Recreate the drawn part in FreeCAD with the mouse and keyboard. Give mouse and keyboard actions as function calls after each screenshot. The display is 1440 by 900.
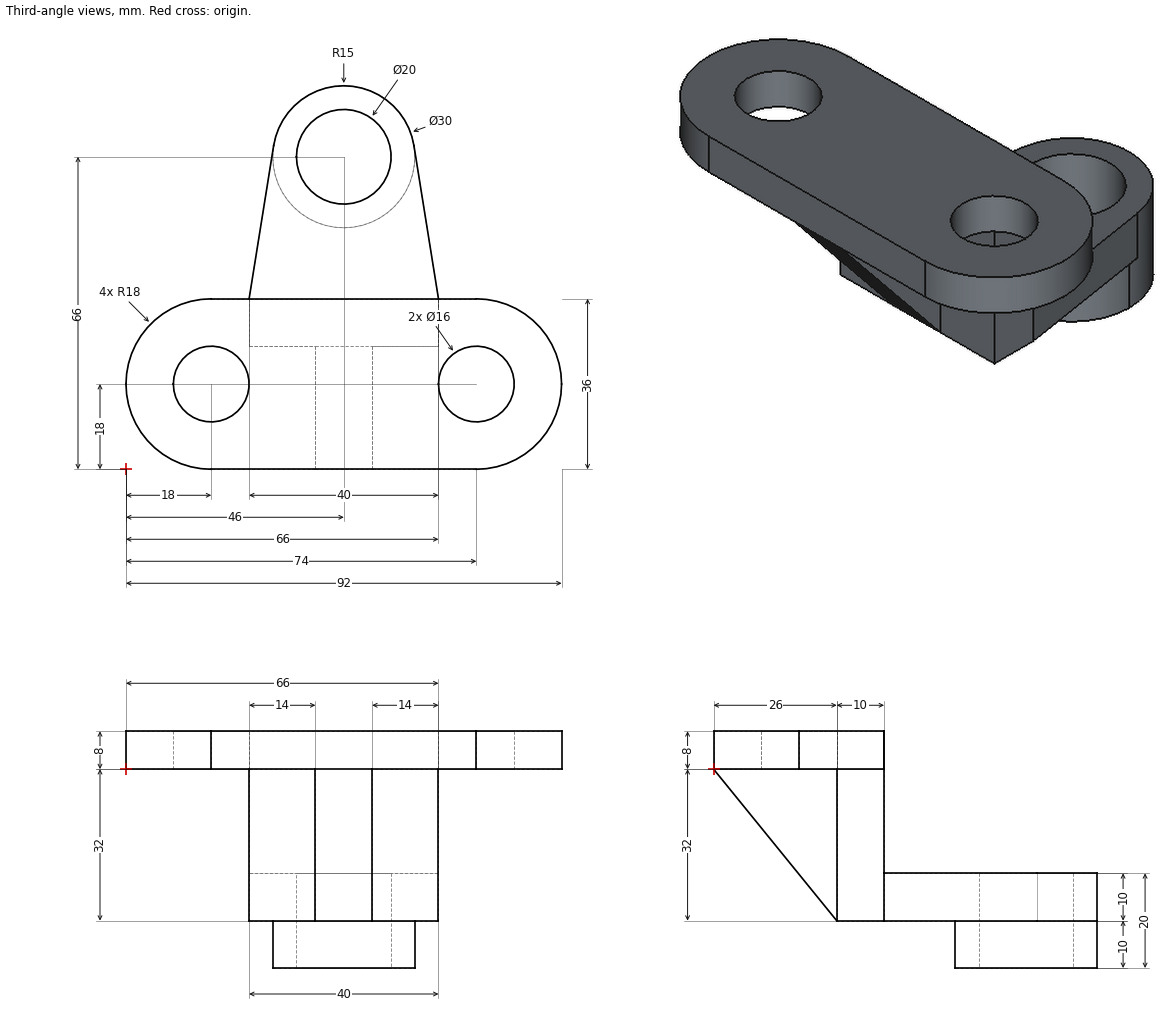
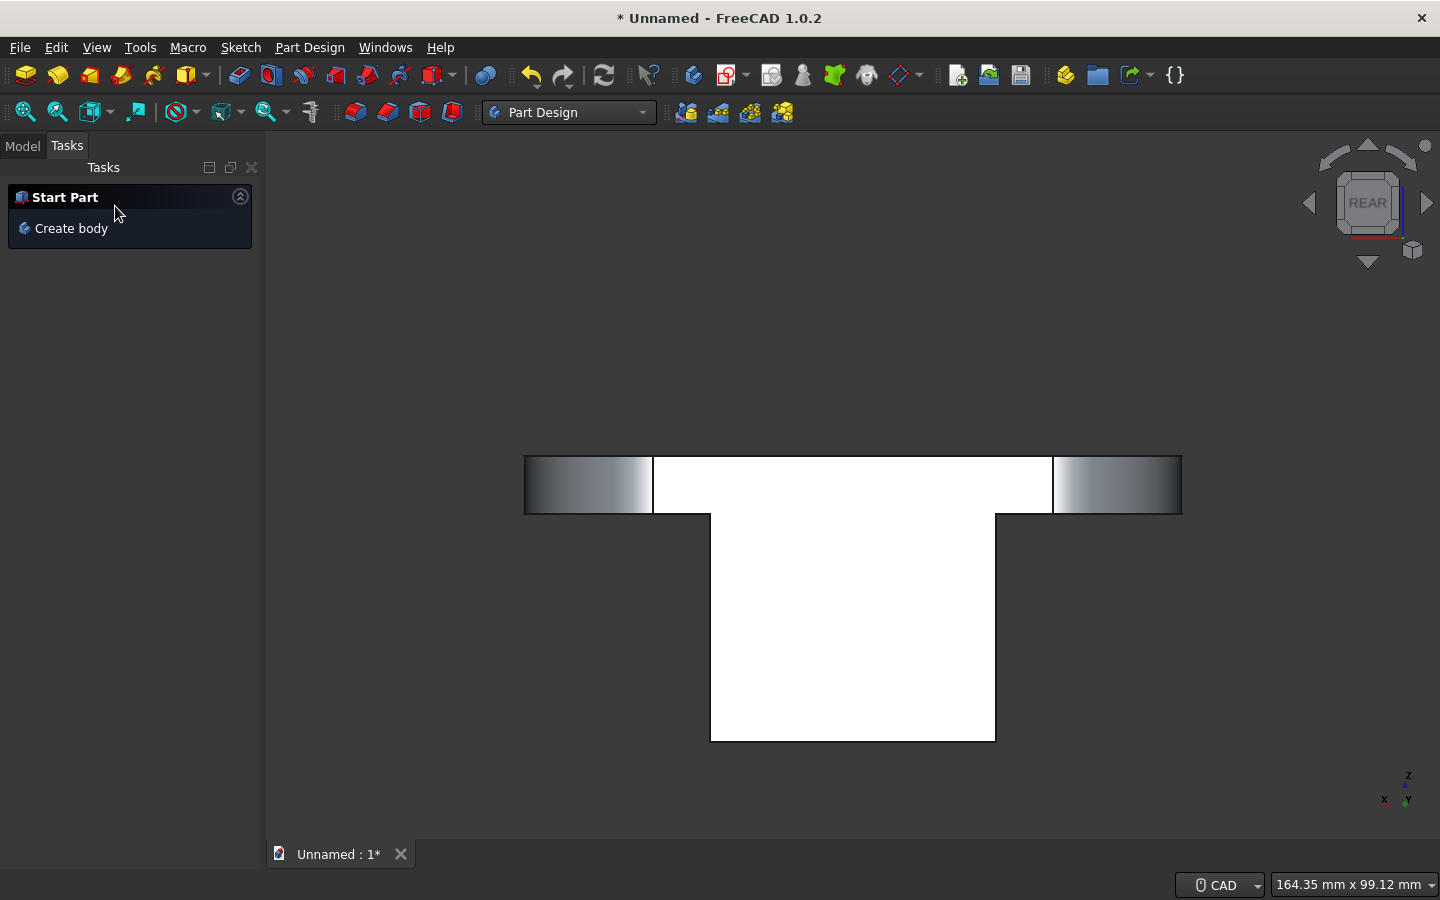
key(5)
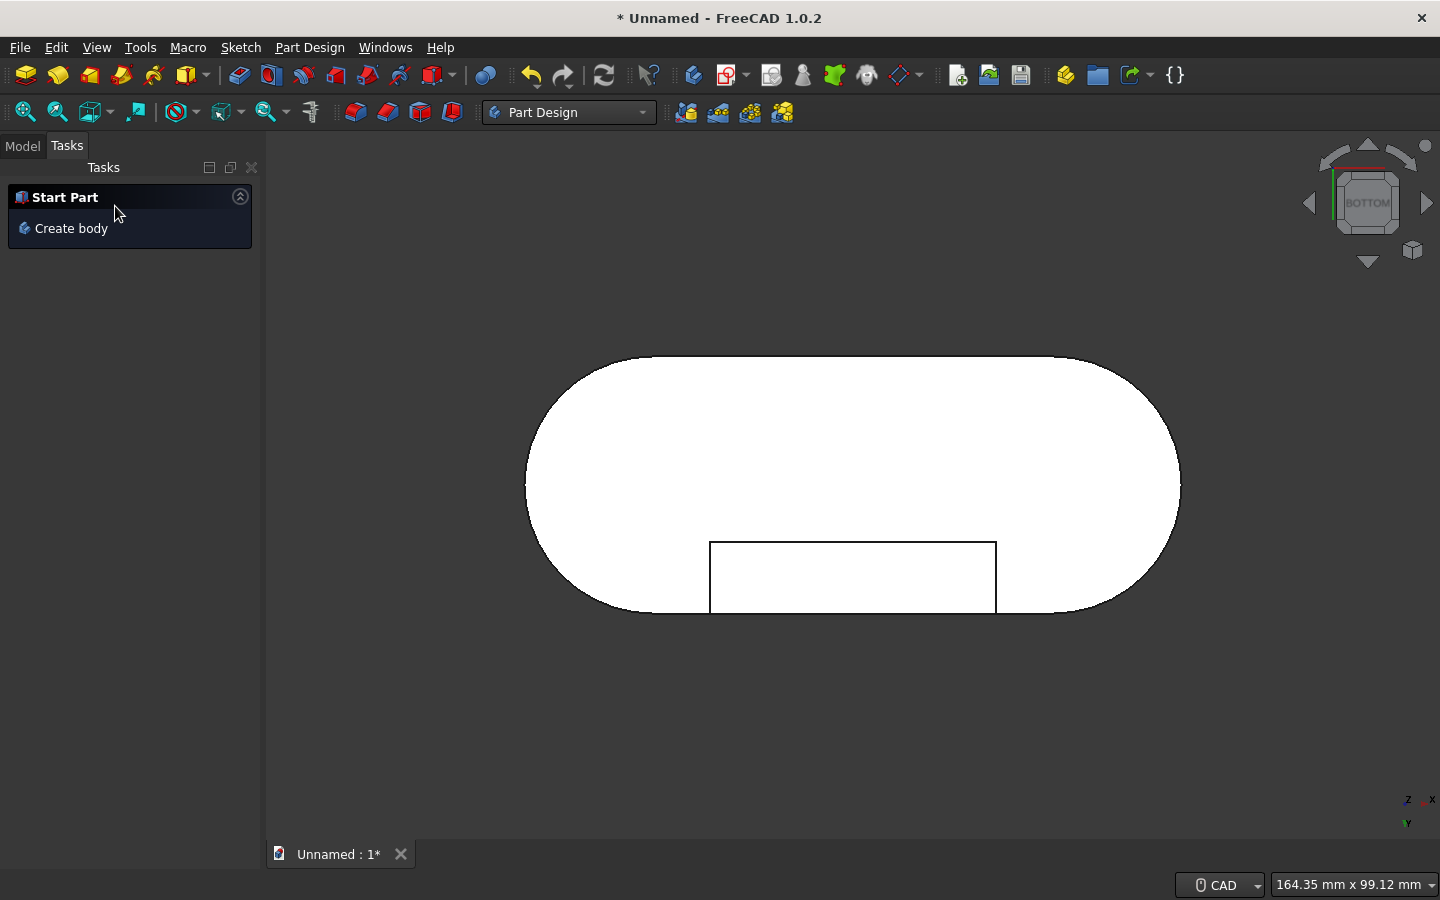
click(935, 577)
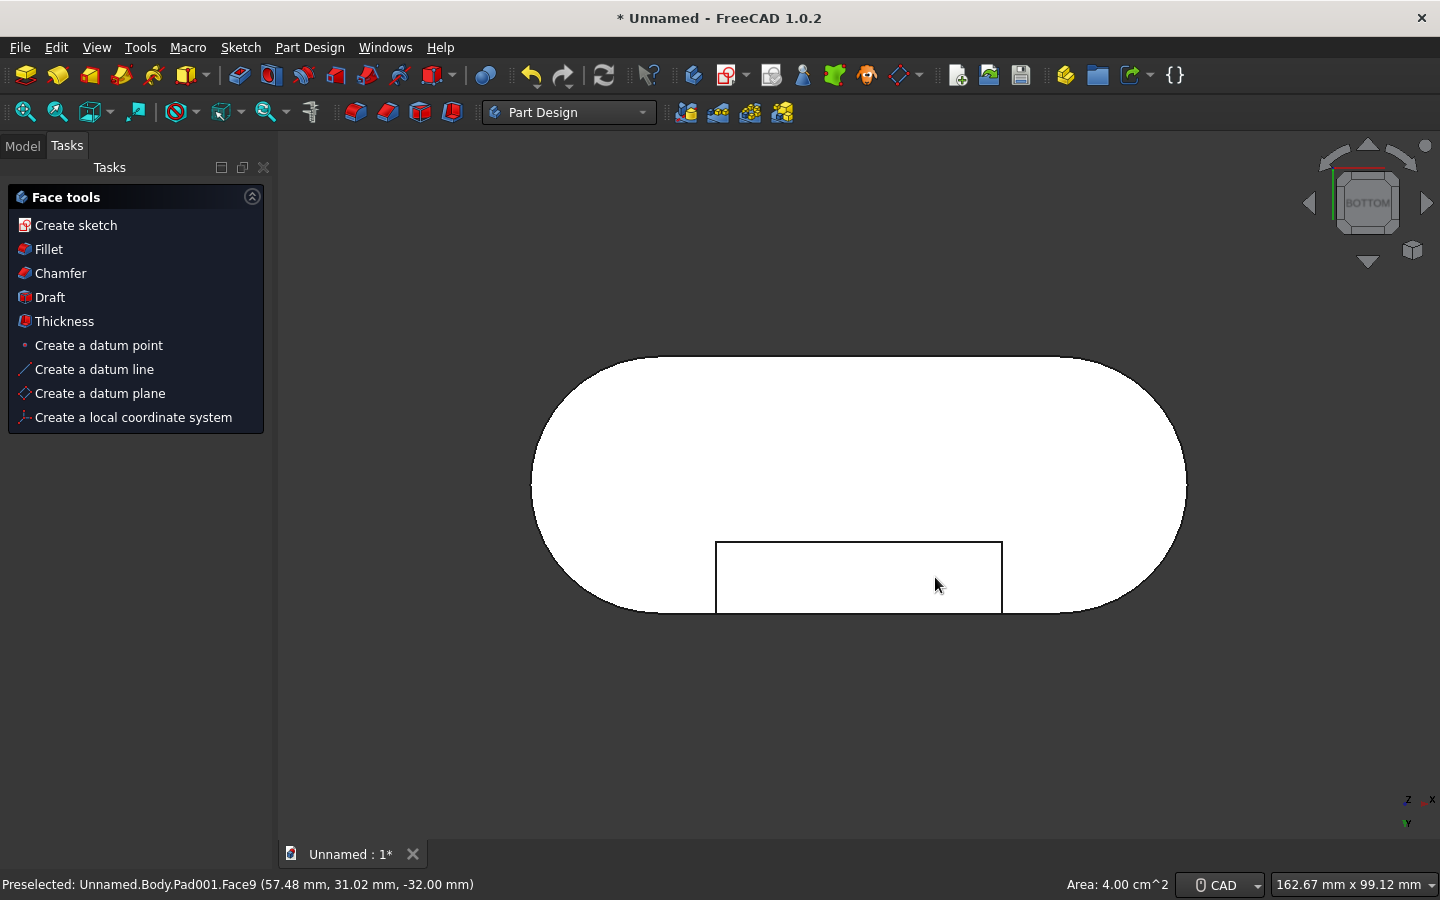
click(726, 76)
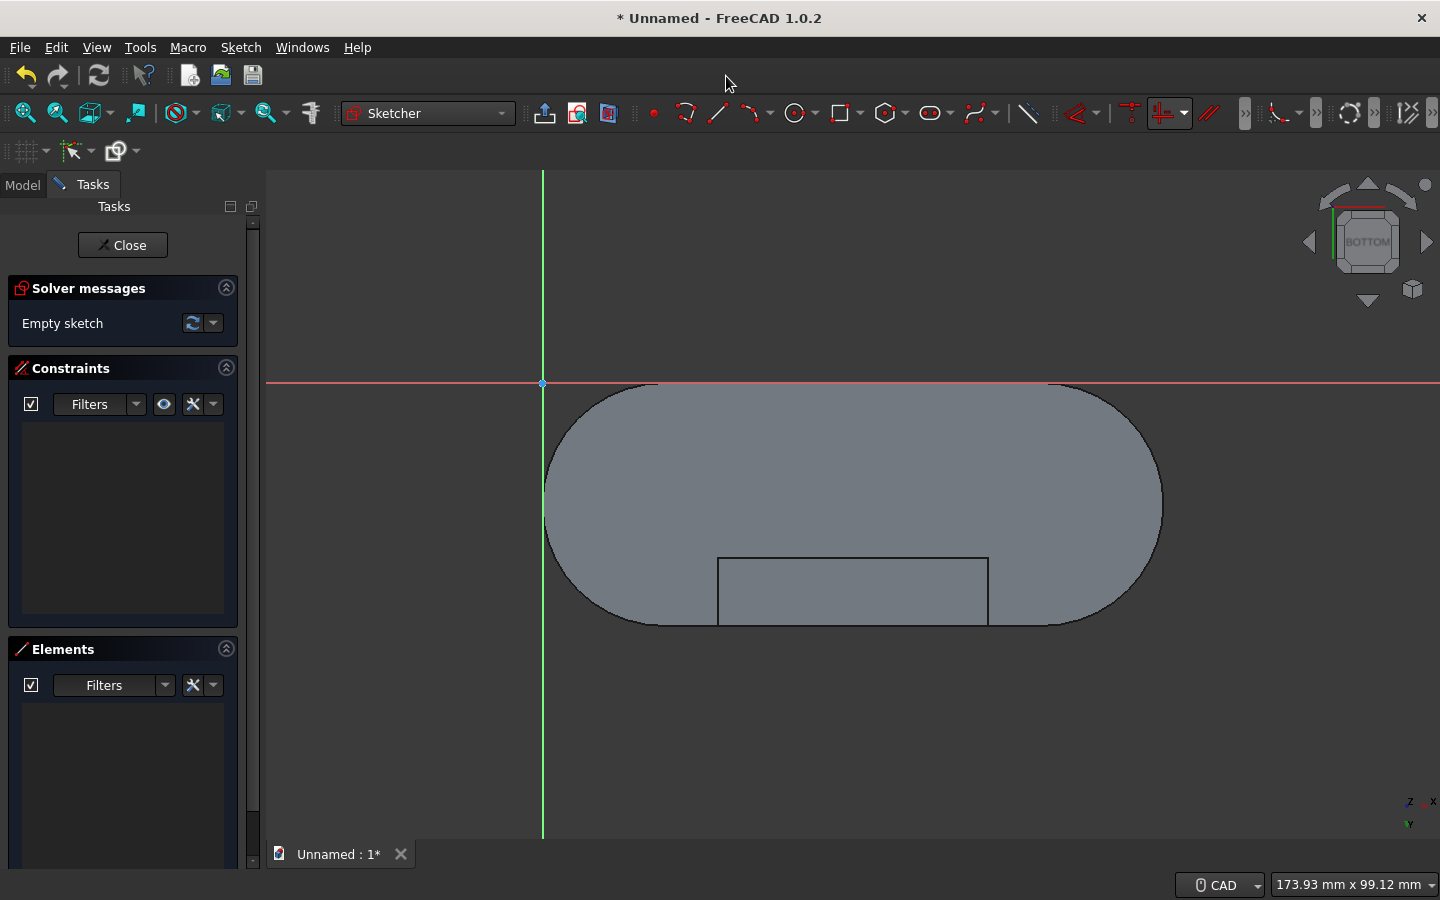
scroll(824, 198, down, 2)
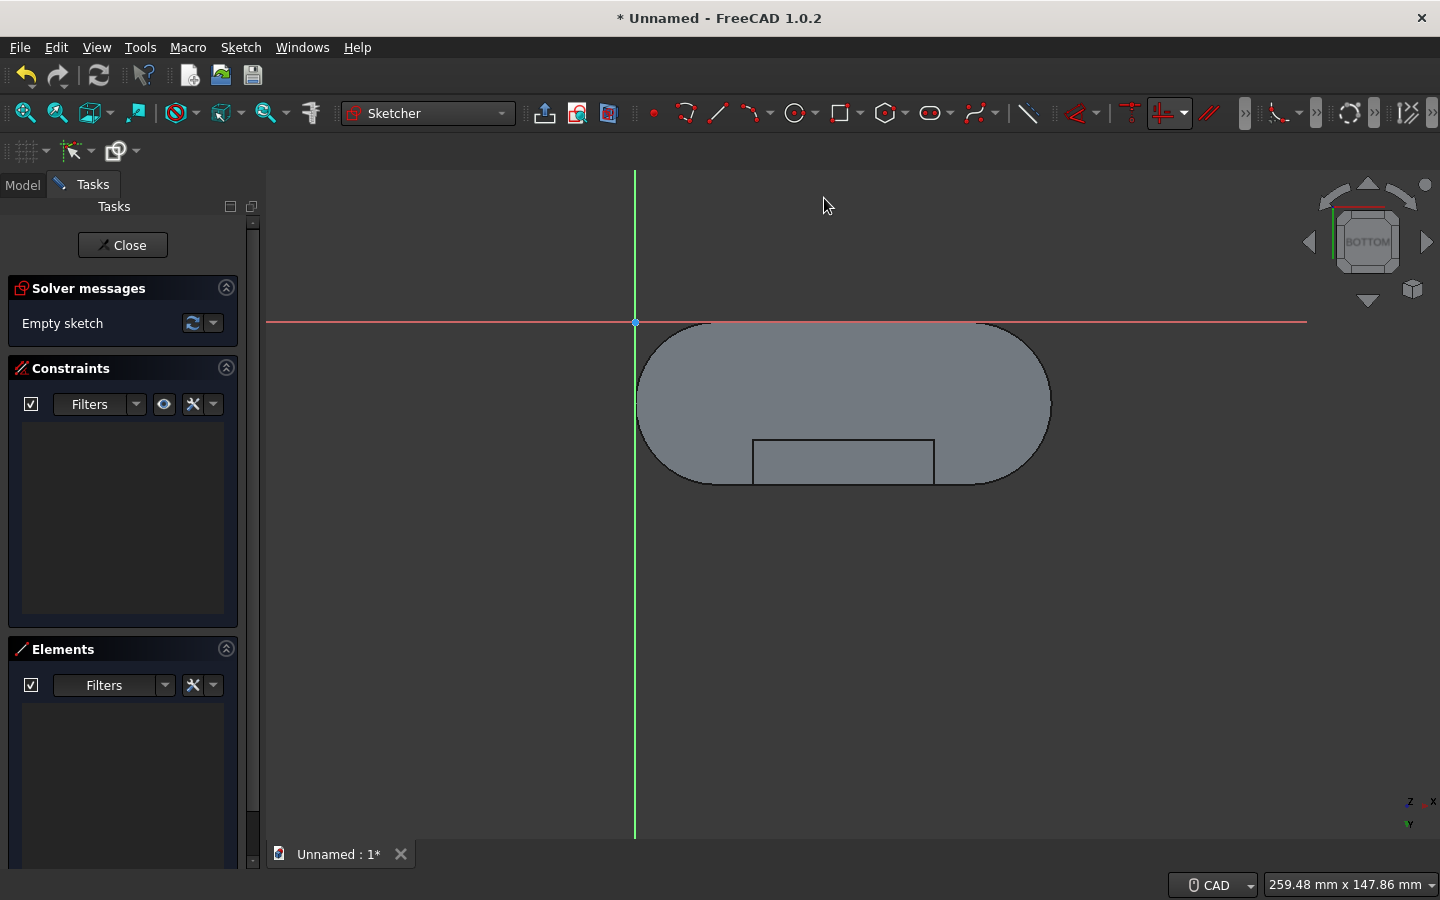
click(686, 114)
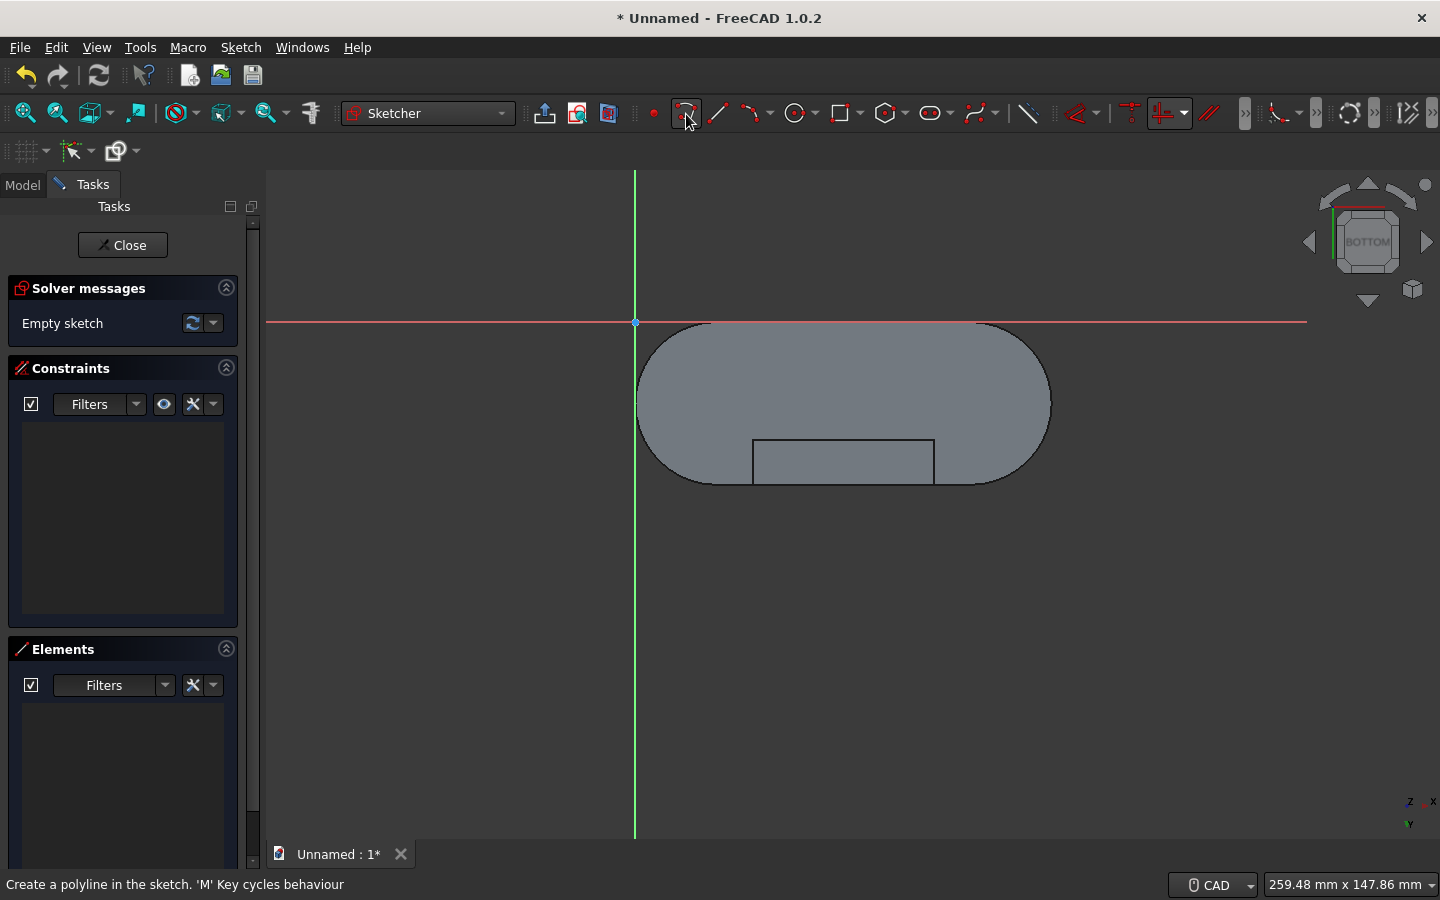
click(911, 631)
click(934, 485)
click(753, 485)
click(777, 631)
right_click(777, 631)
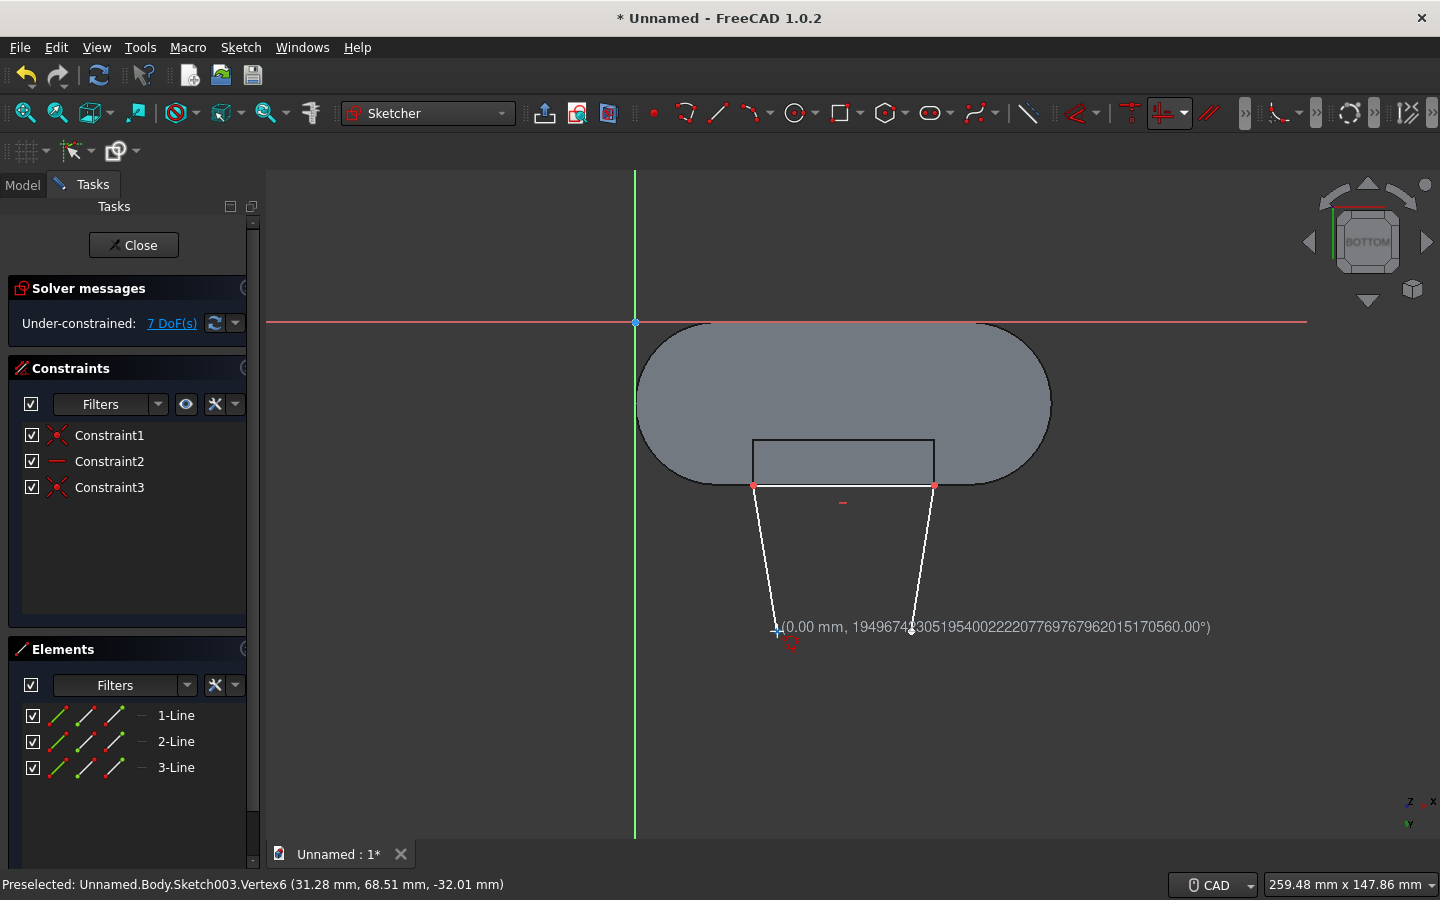
click(750, 114)